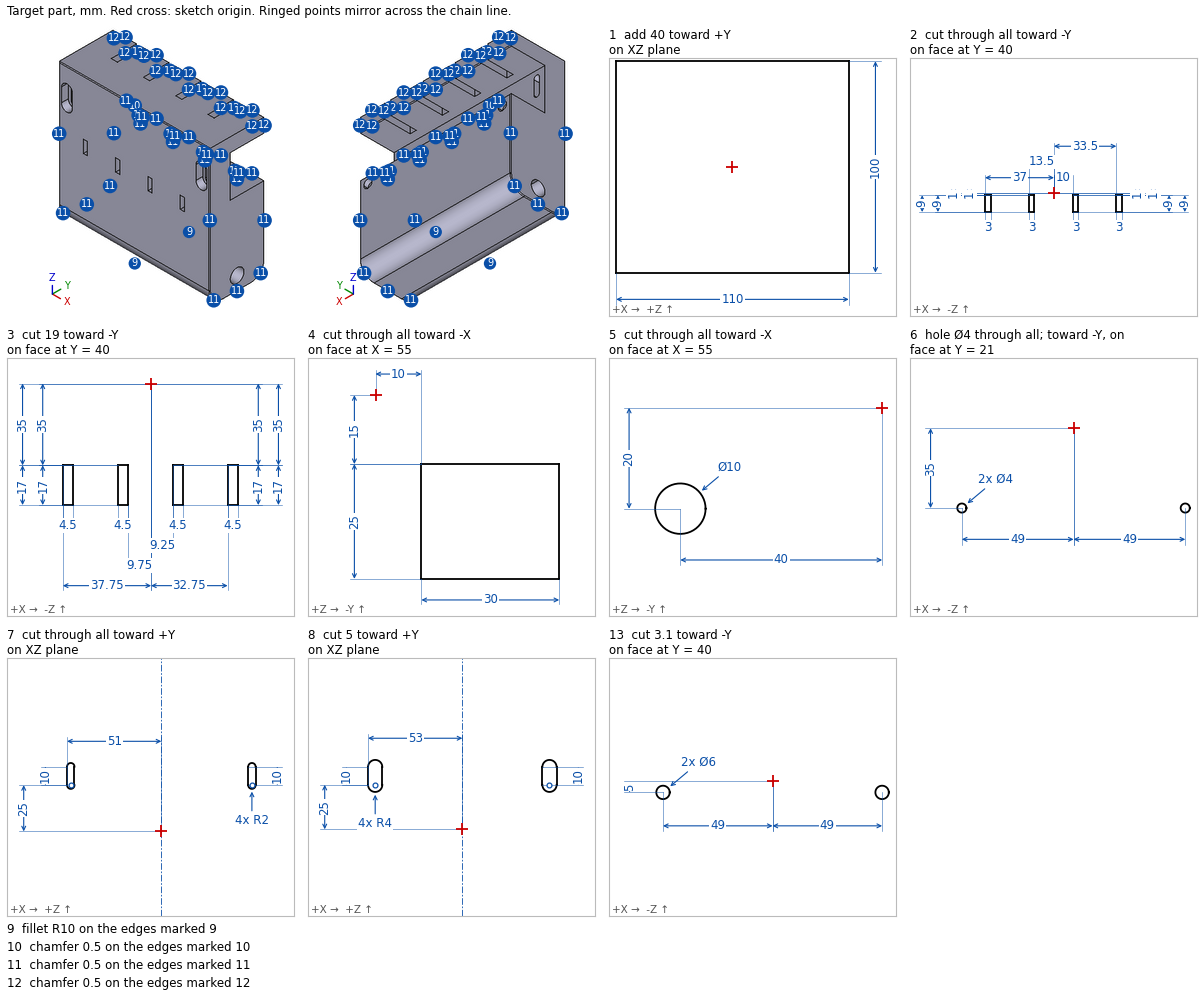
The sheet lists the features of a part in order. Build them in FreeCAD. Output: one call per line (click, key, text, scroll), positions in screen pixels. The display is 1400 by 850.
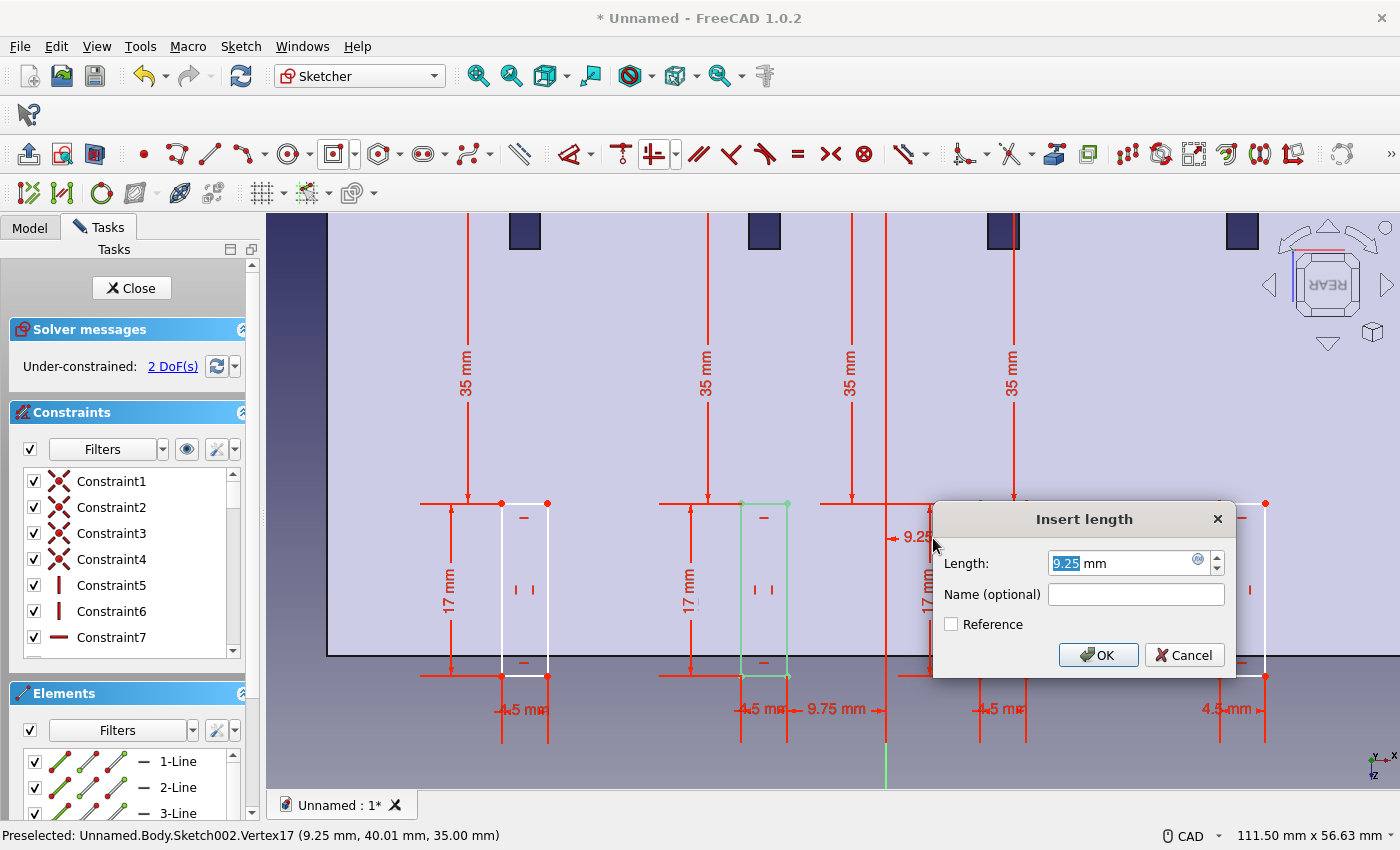
text(9.25)
key(Return)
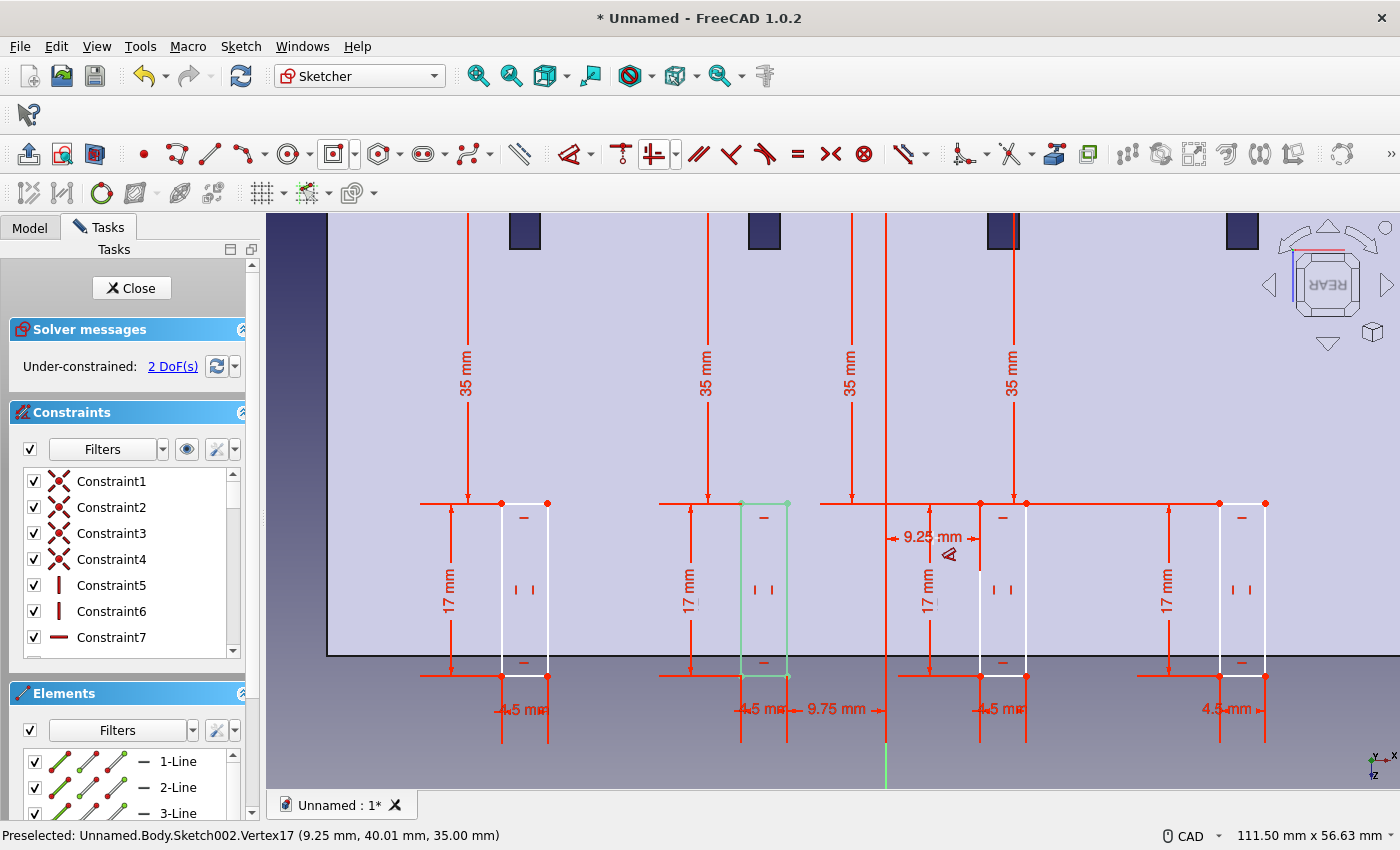
click(502, 504)
click(694, 538)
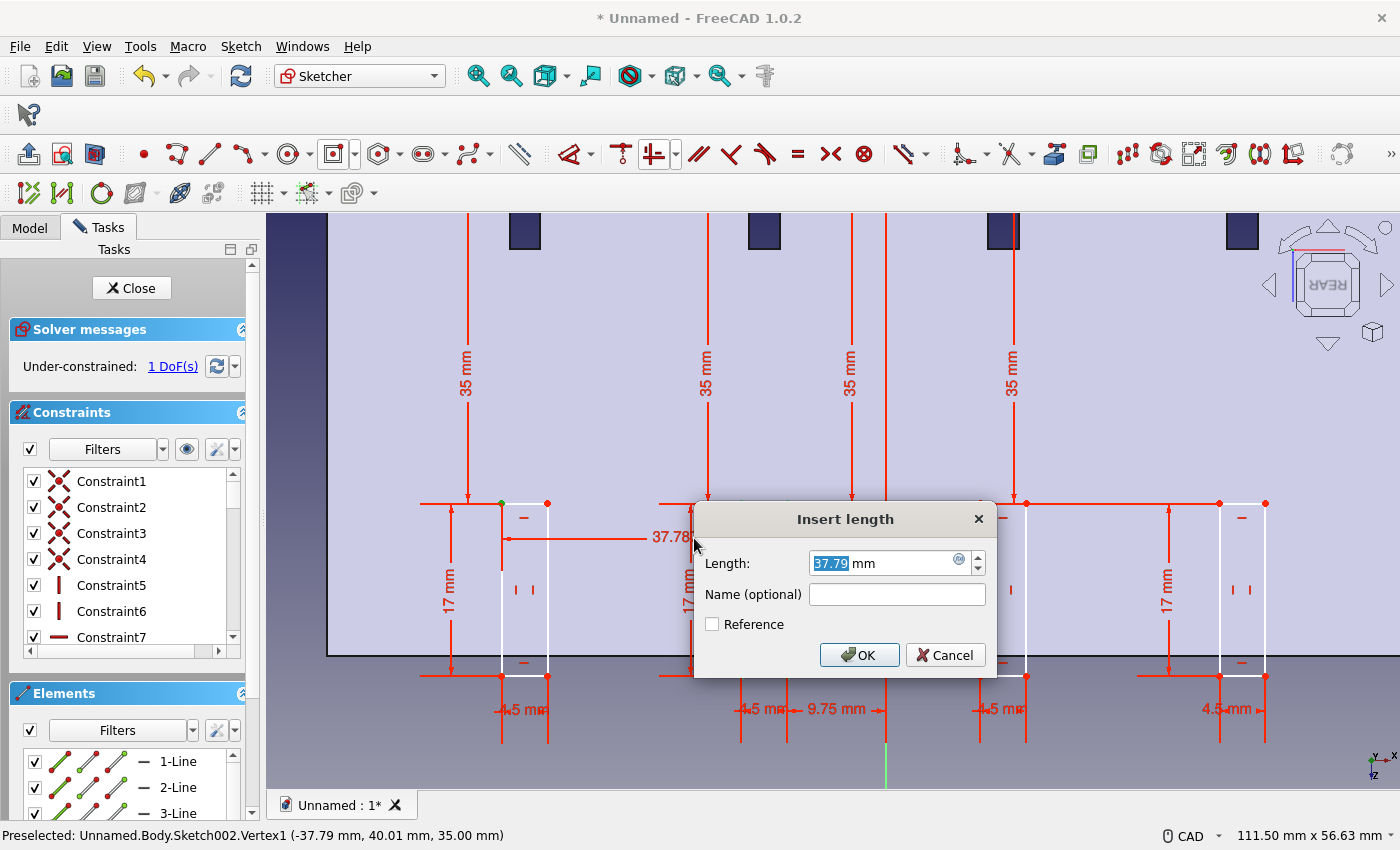
text(37.75)
key(Return)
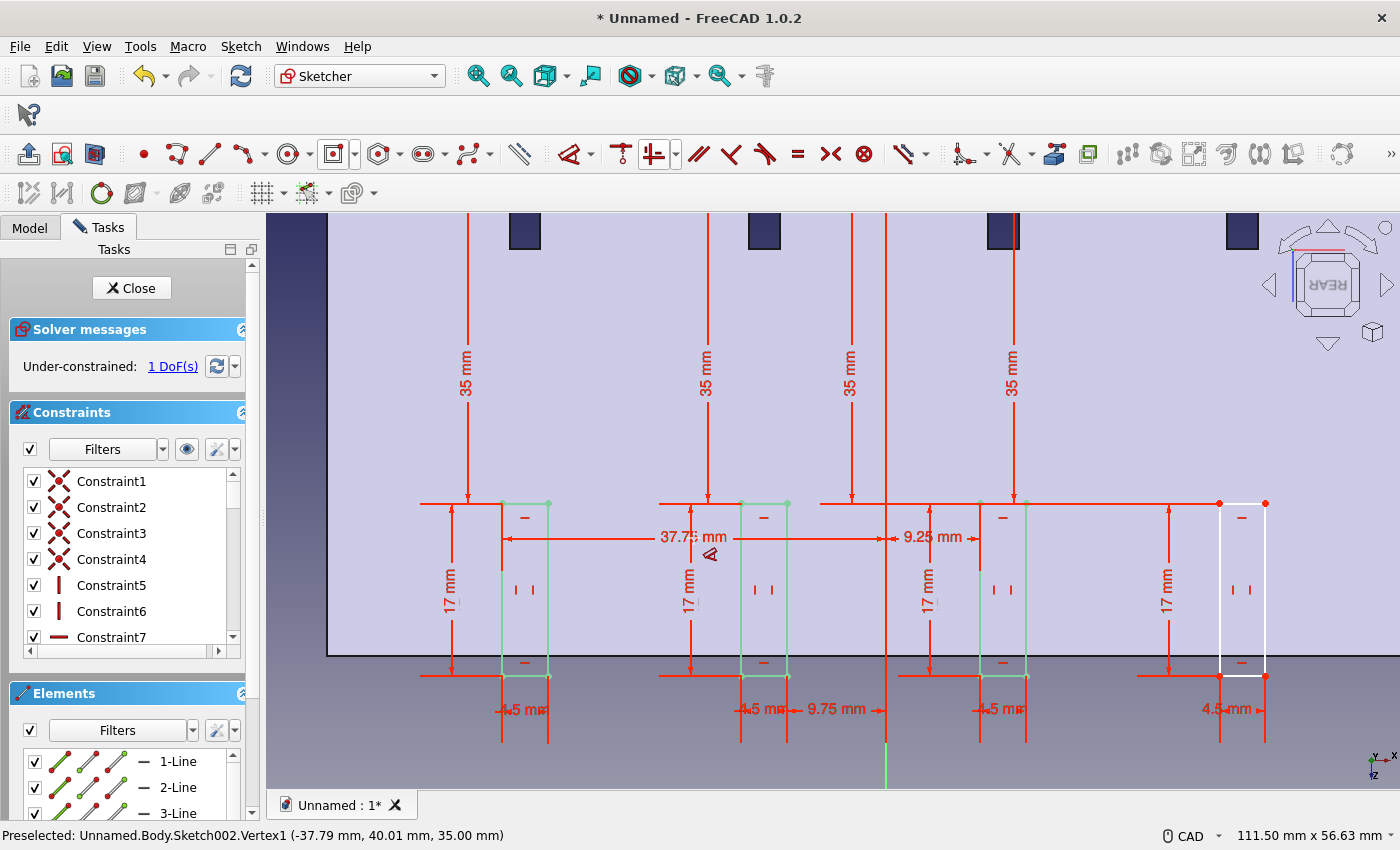
click(1220, 504)
click(1053, 538)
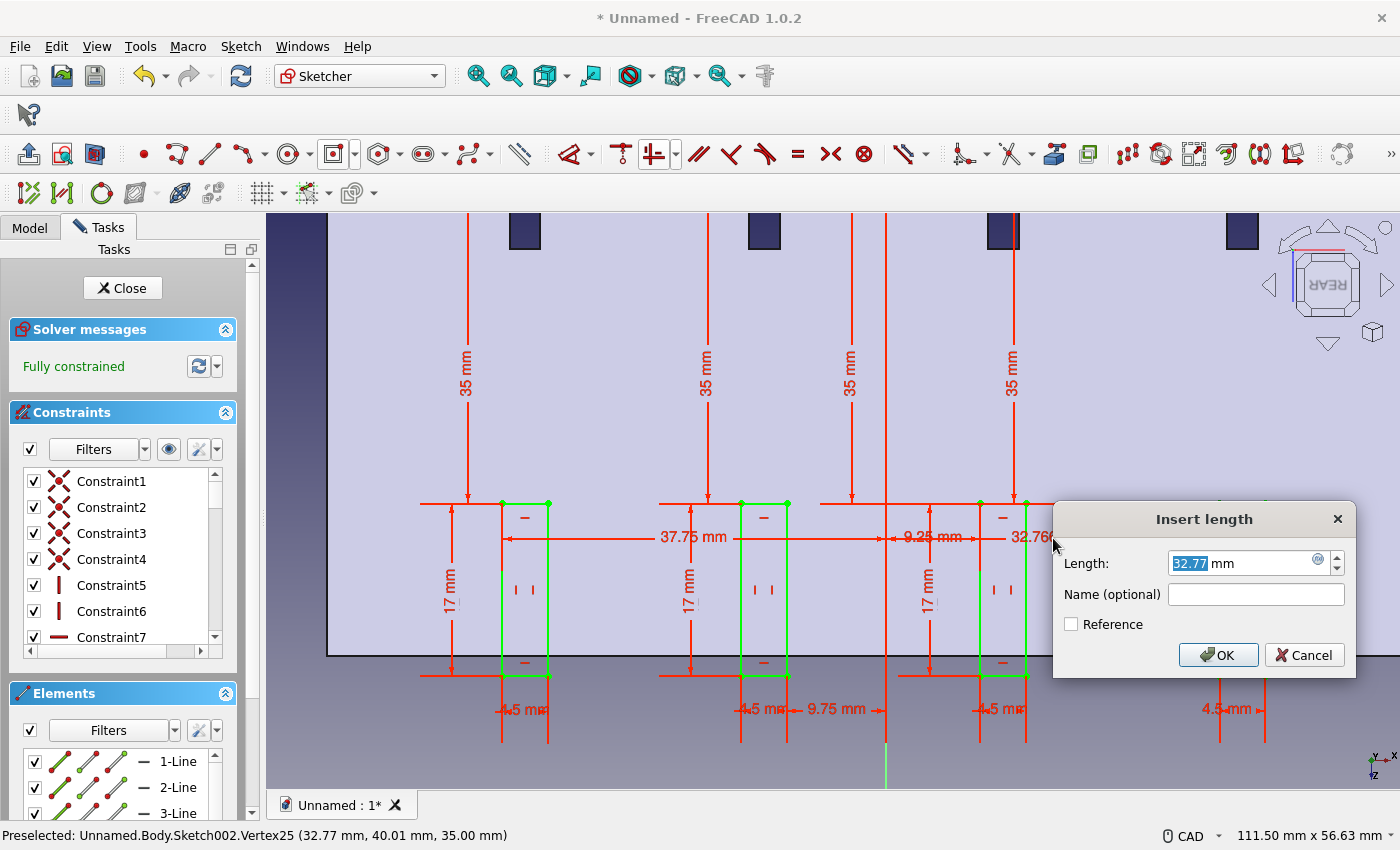
text(32.75)
key(Return)
key(Escape)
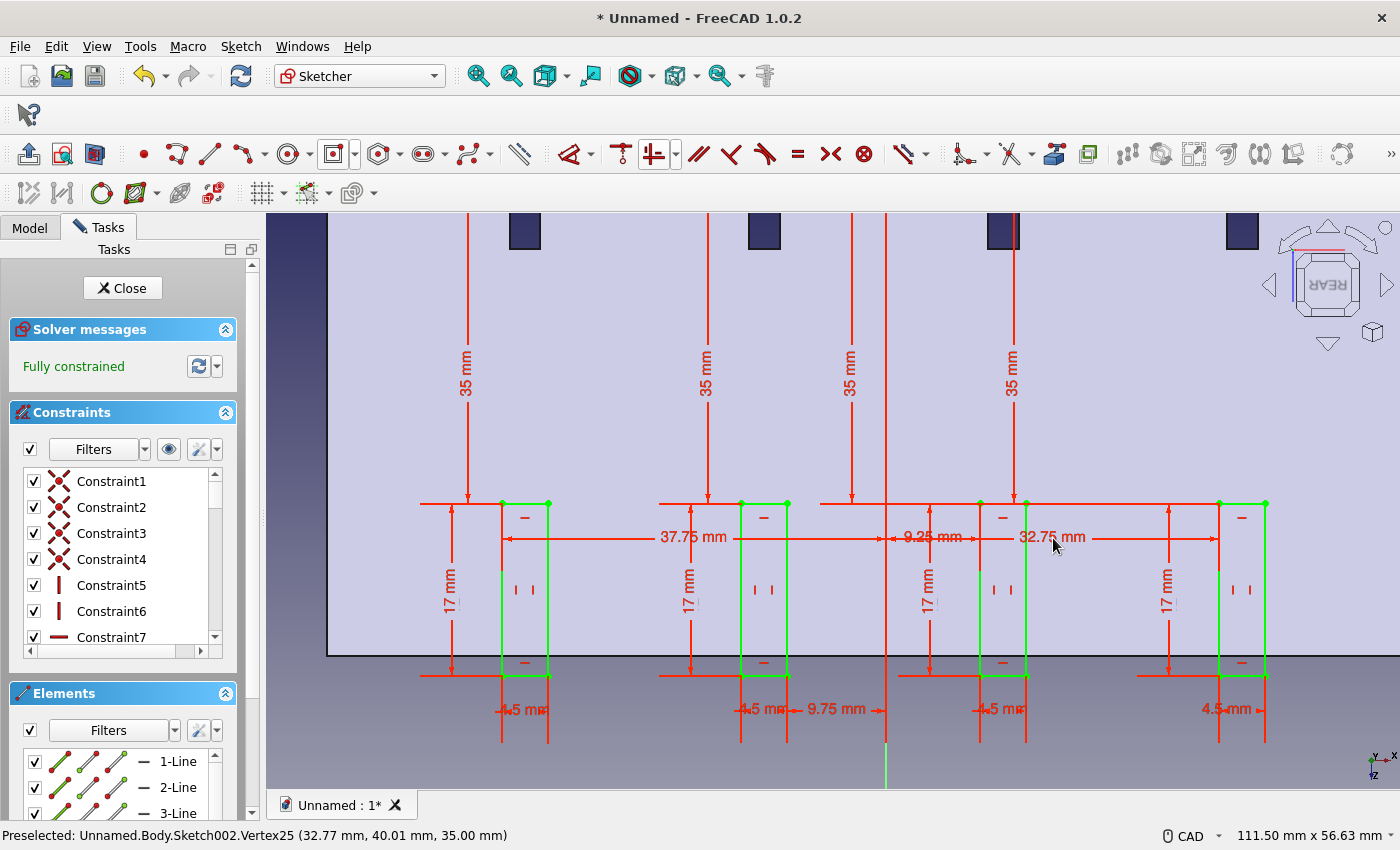
click(123, 288)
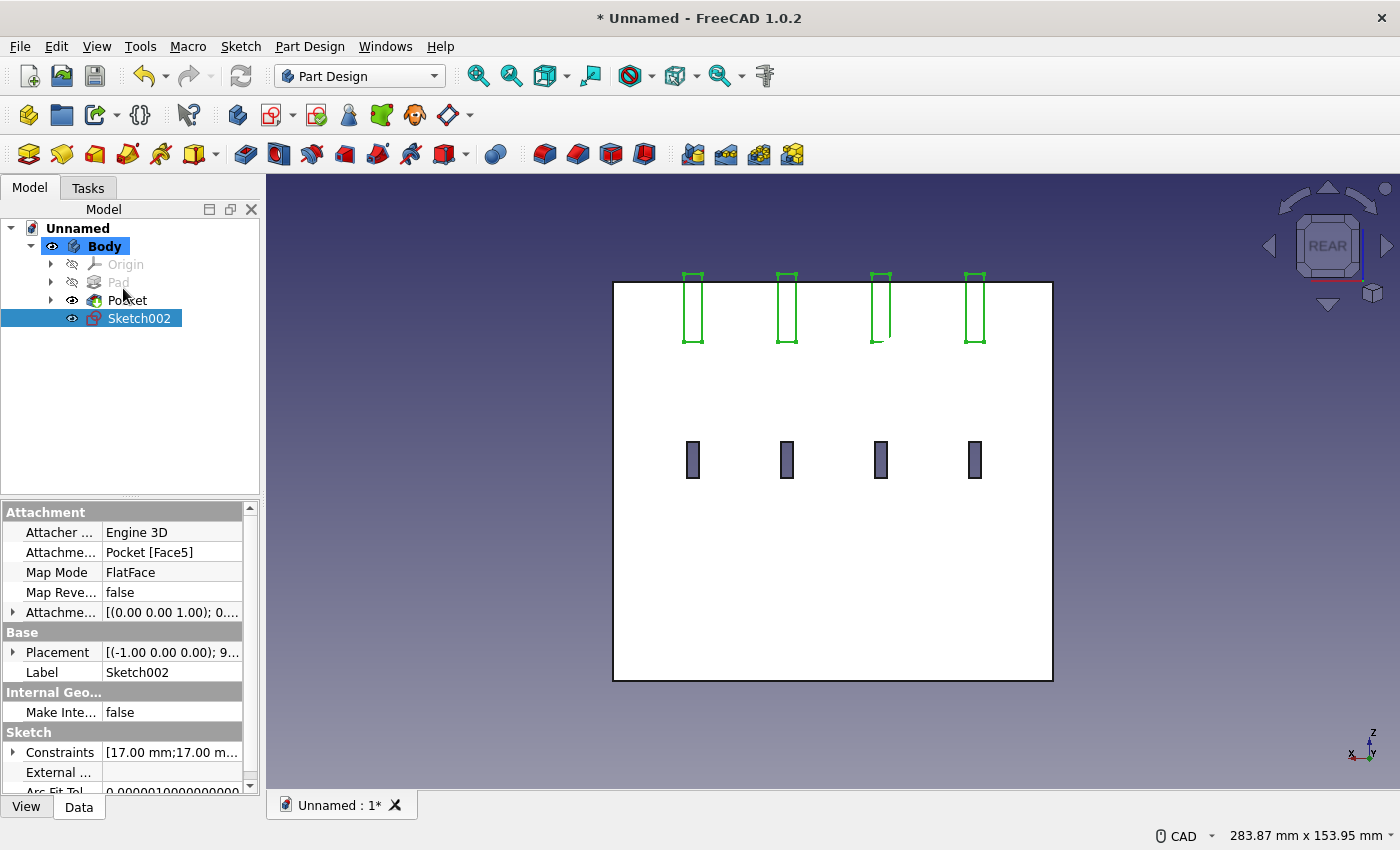
click(246, 154)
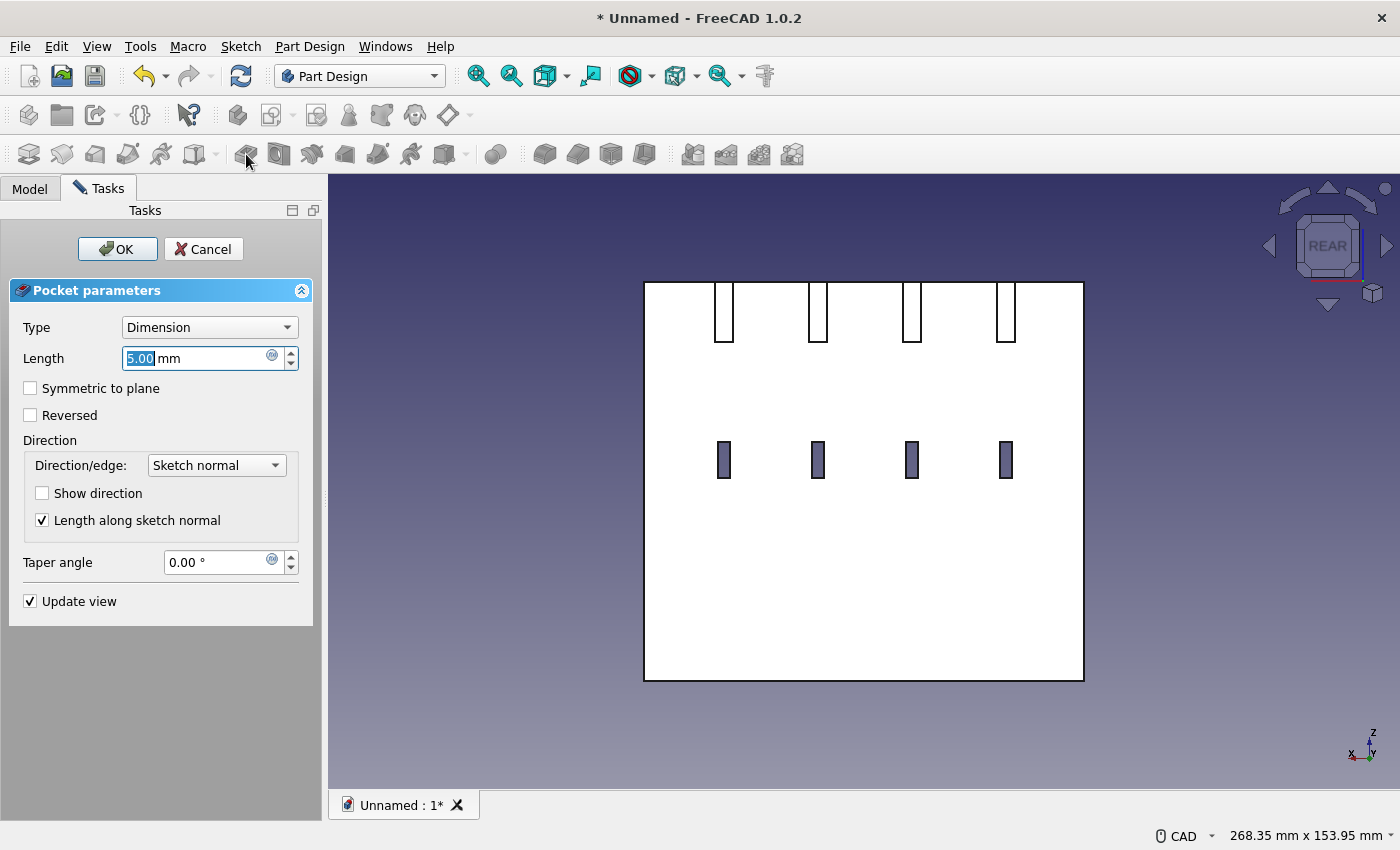
text(19)
key(Tab)